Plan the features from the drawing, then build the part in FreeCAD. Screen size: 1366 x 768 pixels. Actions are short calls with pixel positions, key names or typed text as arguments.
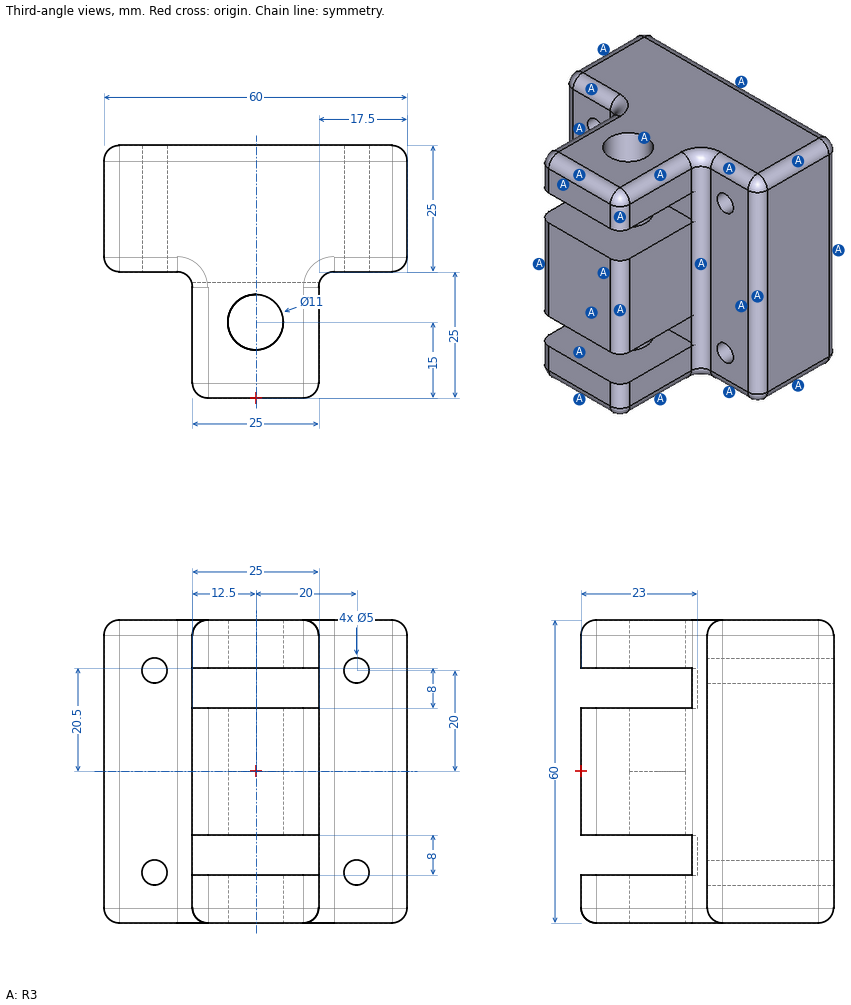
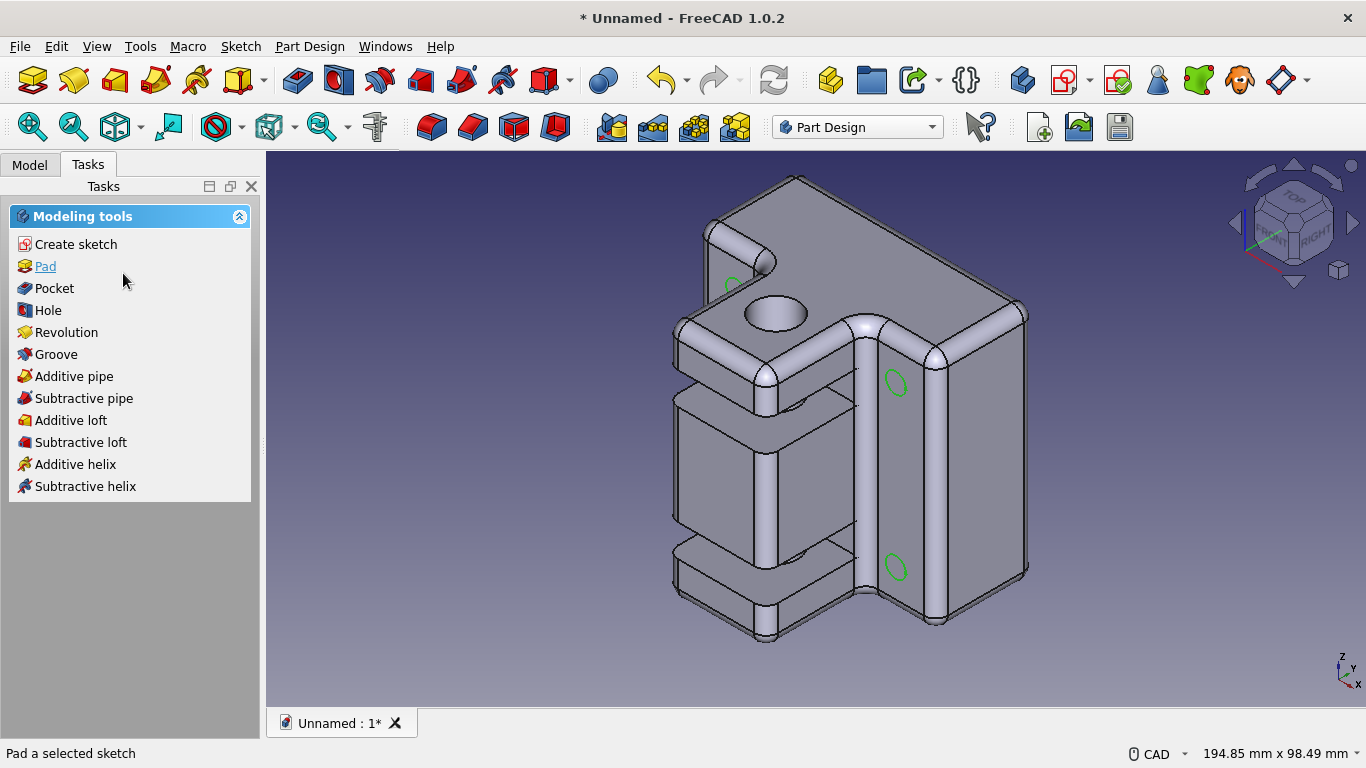
click(298, 80)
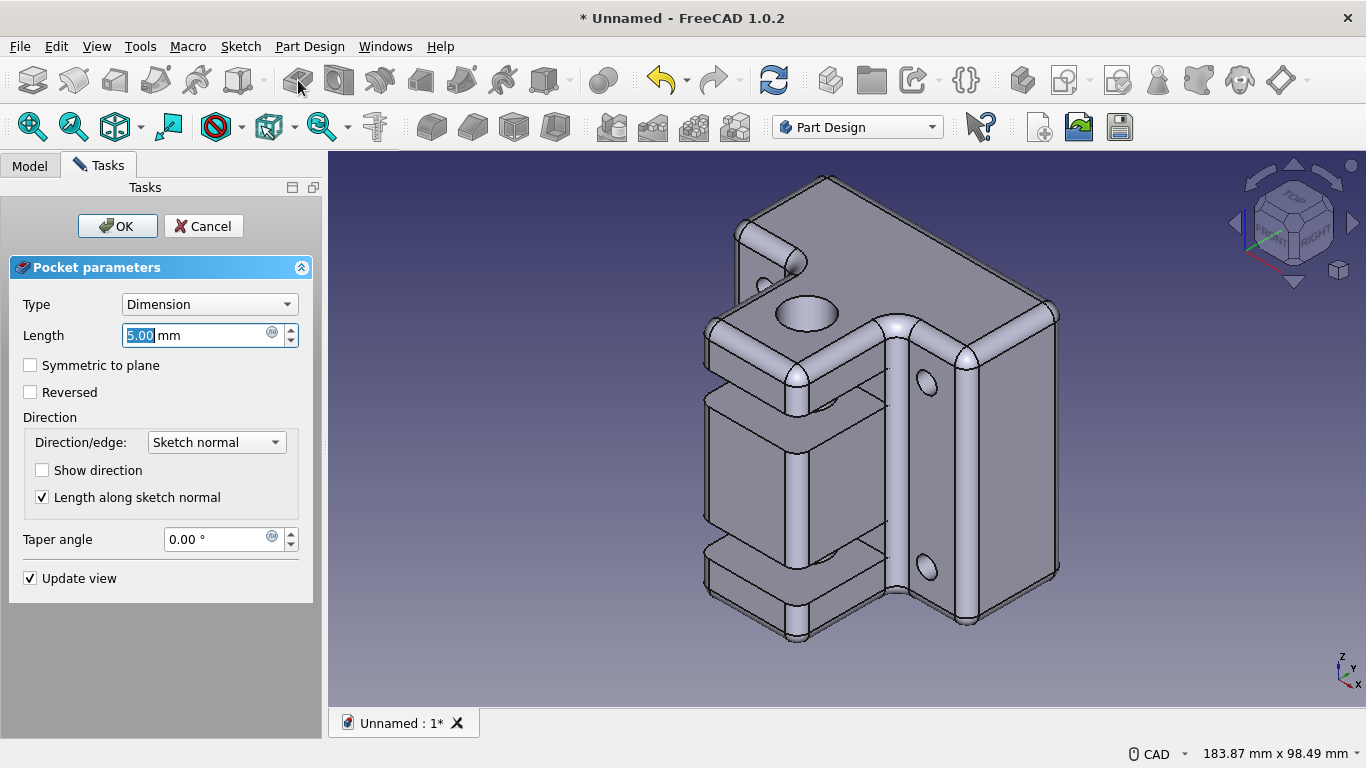
click(210, 304)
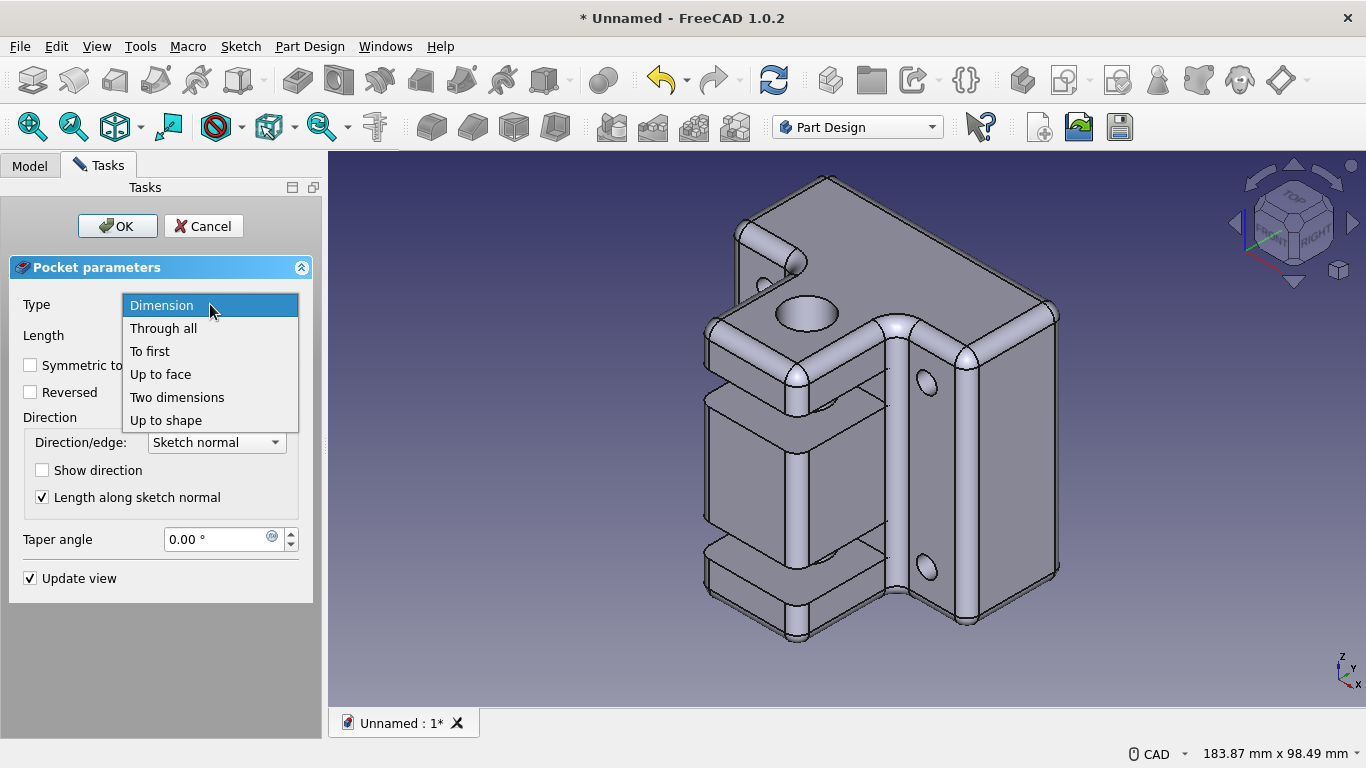
click(208, 328)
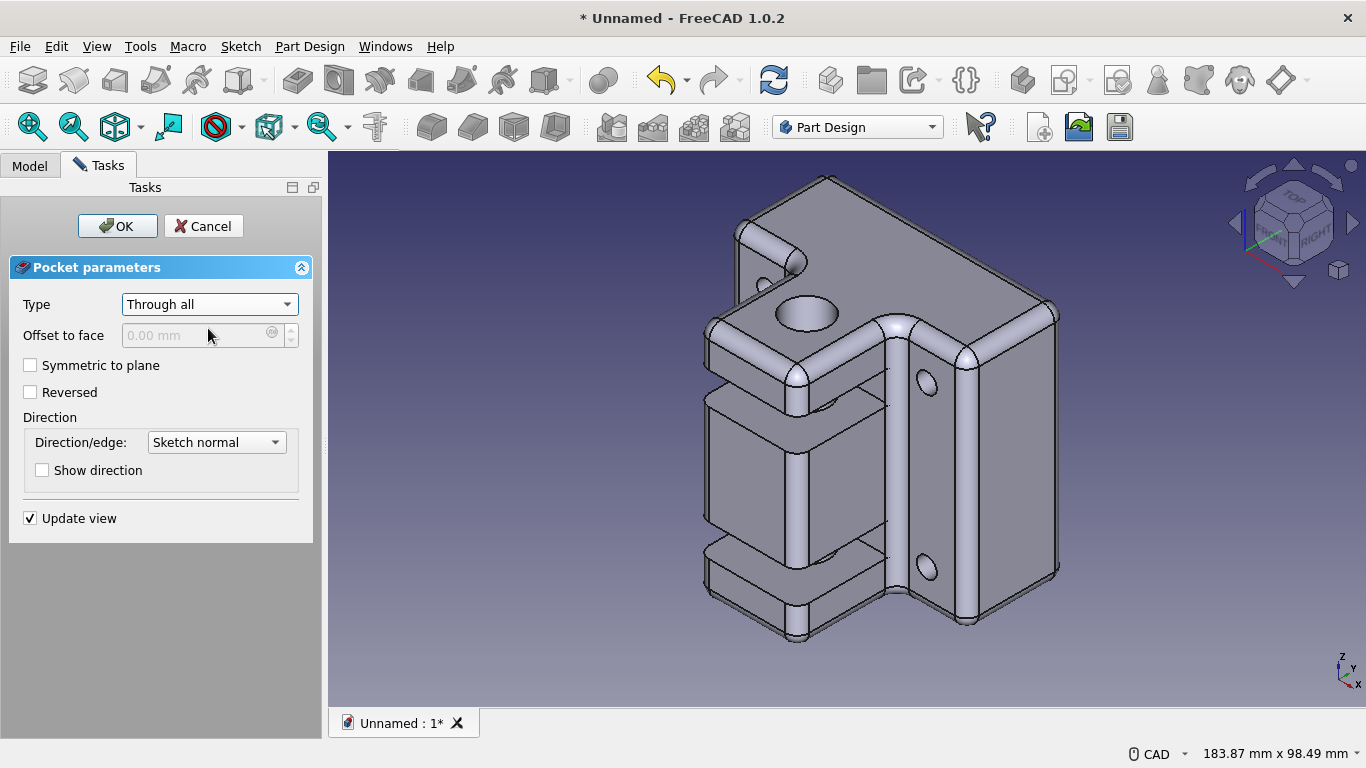
click(118, 226)